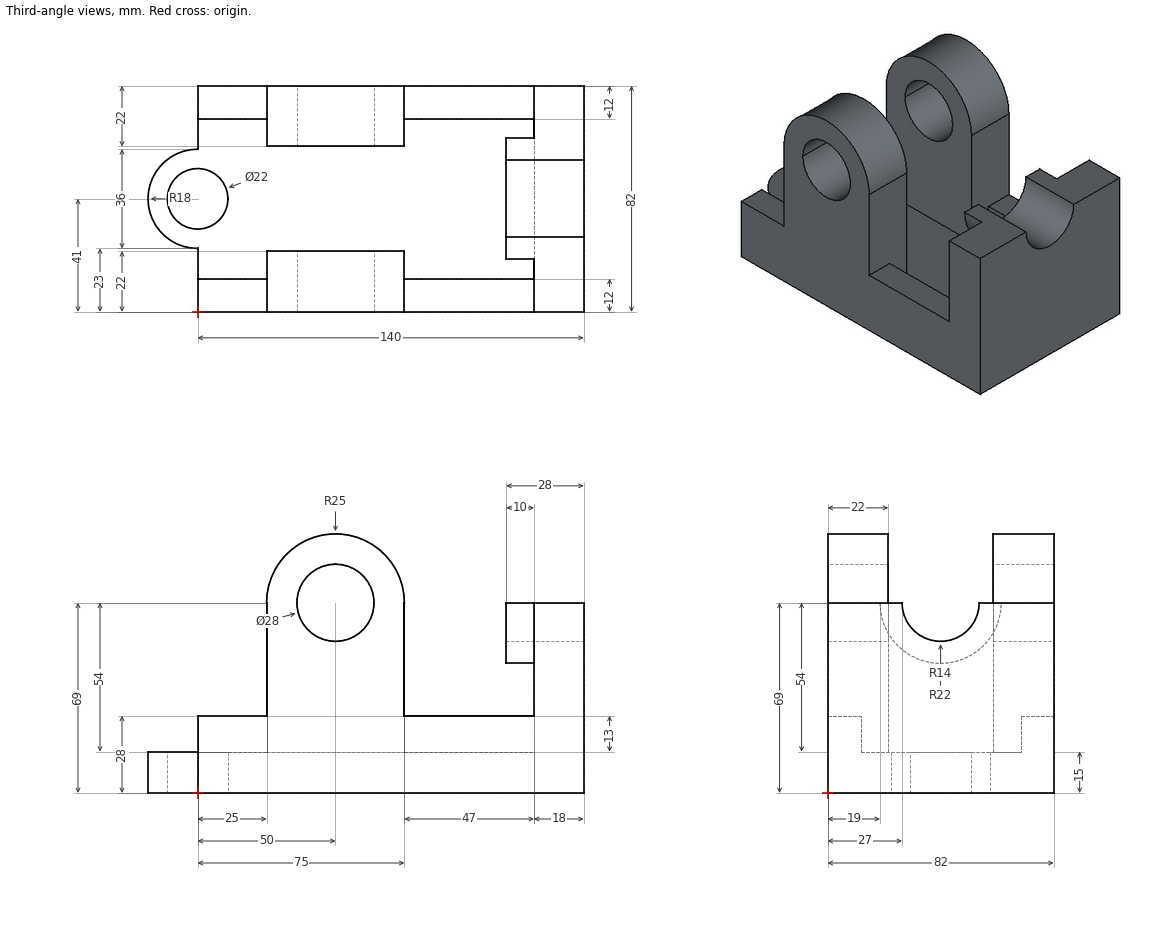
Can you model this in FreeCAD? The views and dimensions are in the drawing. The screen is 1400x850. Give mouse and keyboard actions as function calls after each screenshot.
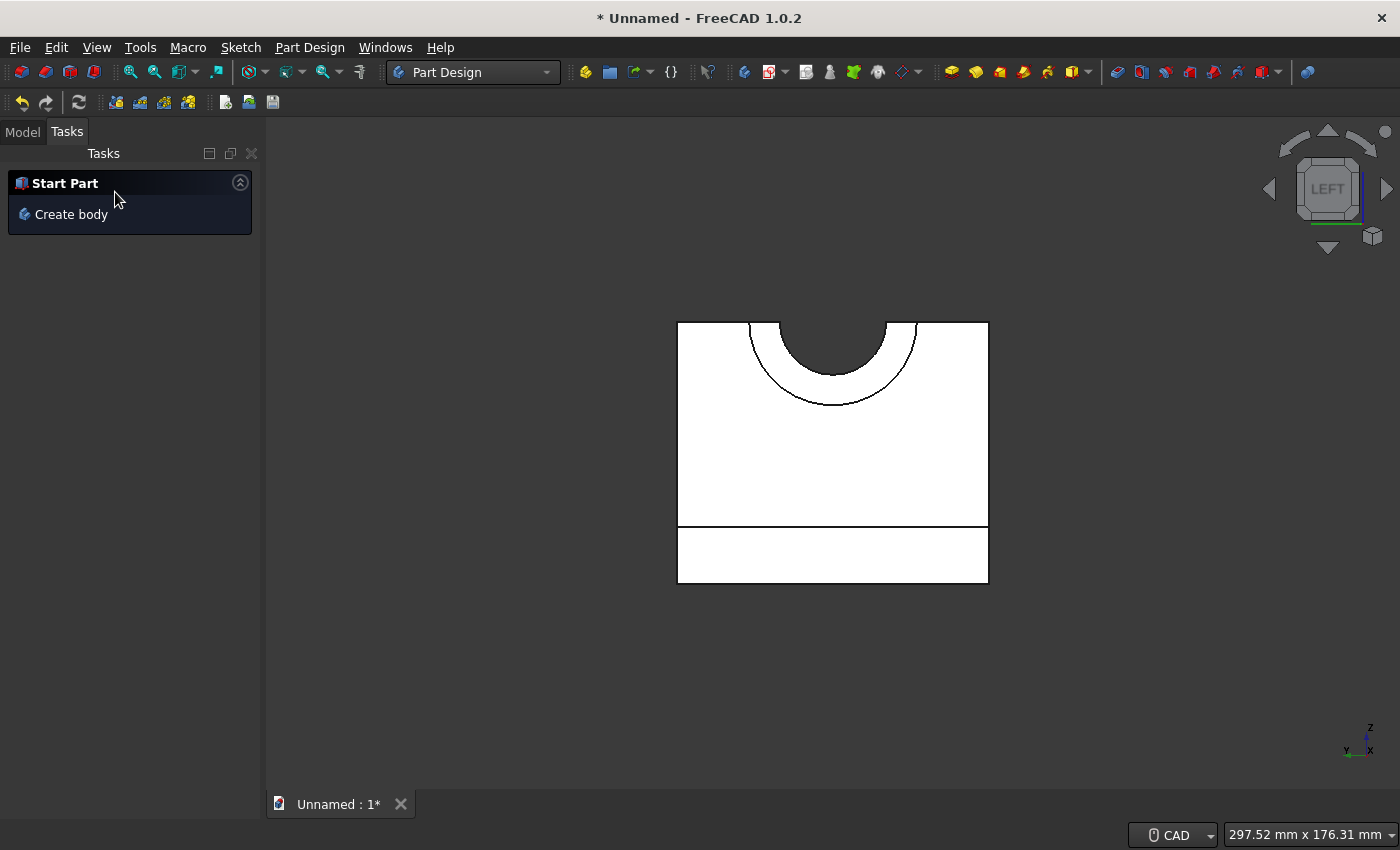
click(132, 72)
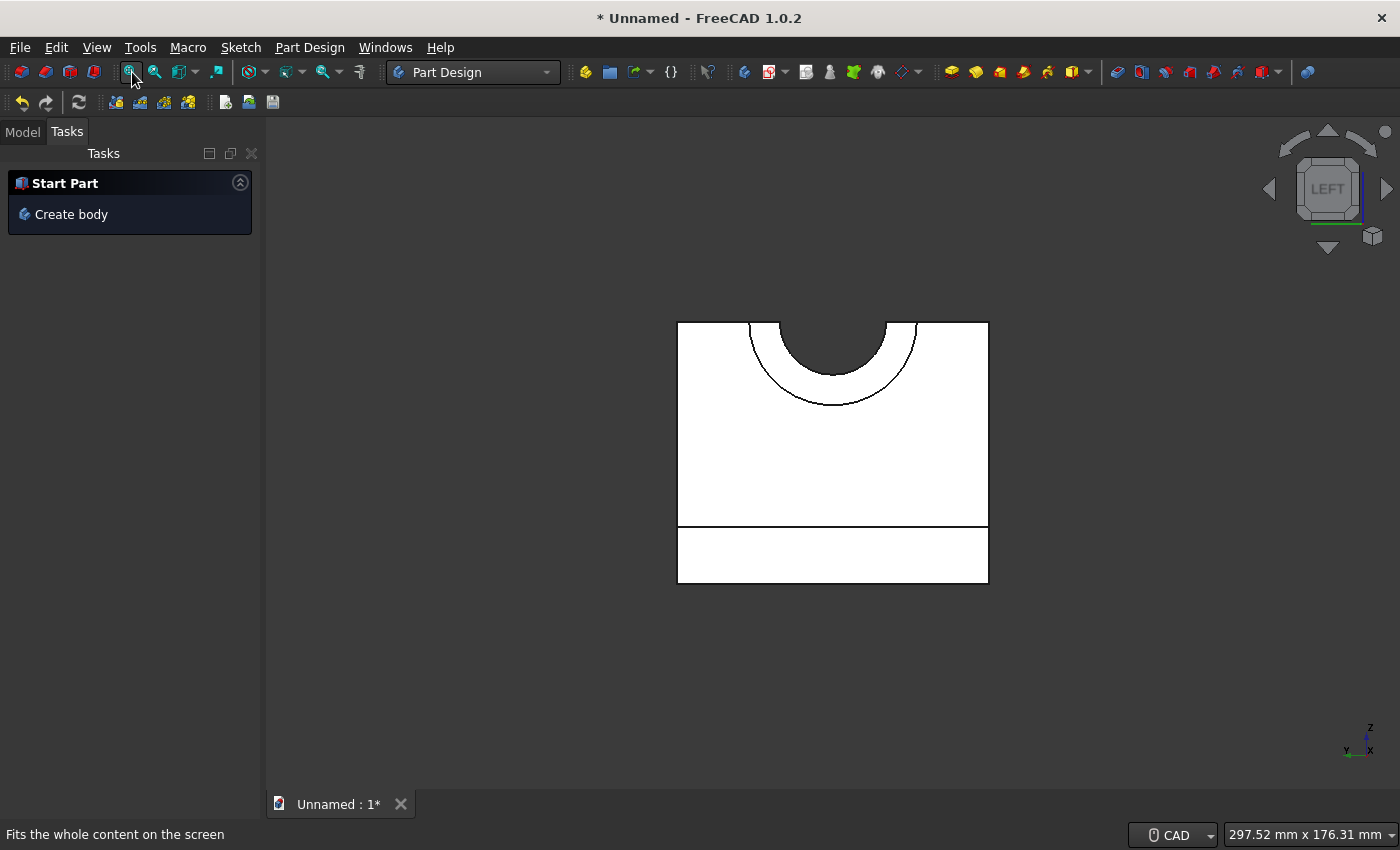
click(770, 72)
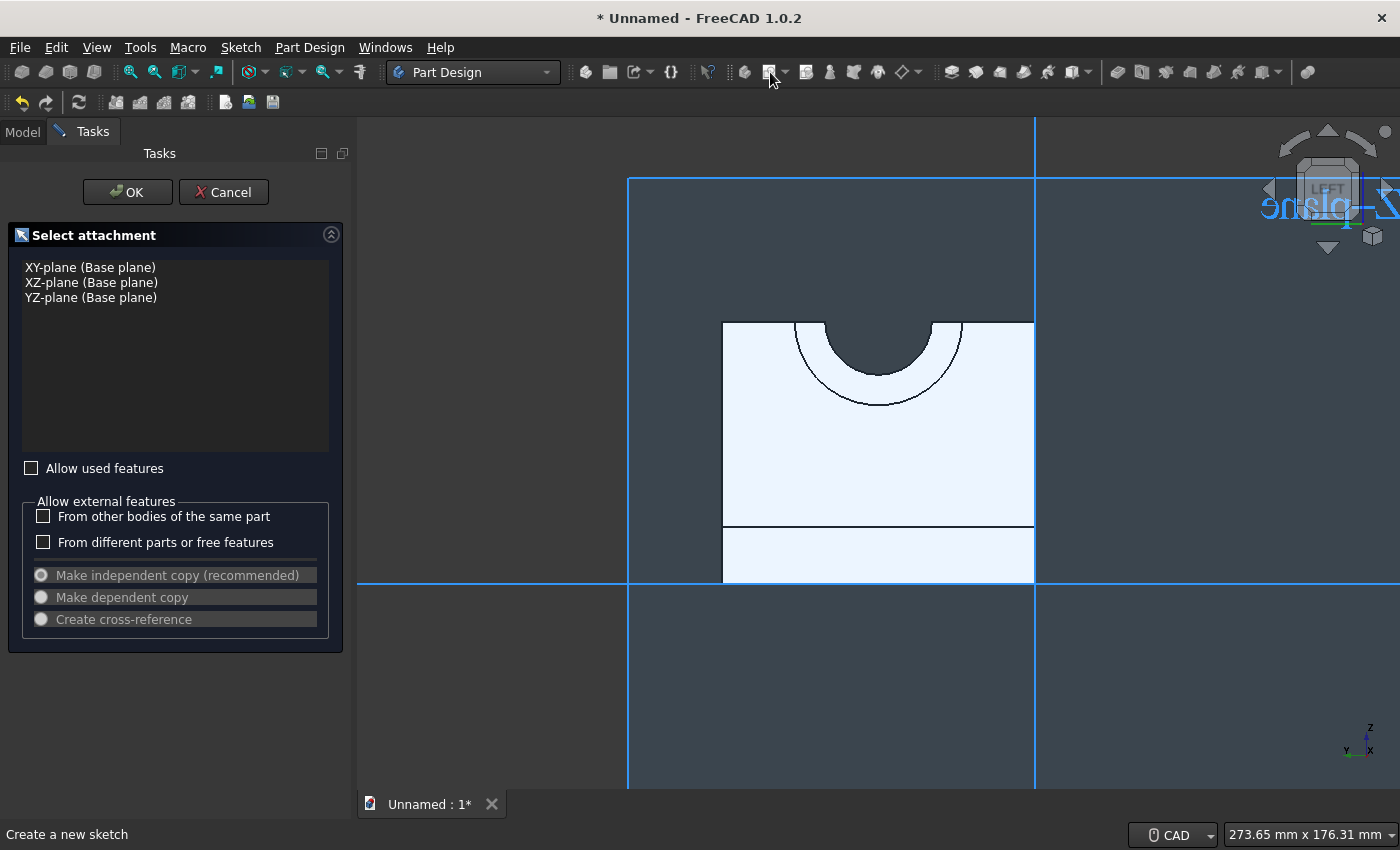
click(82, 282)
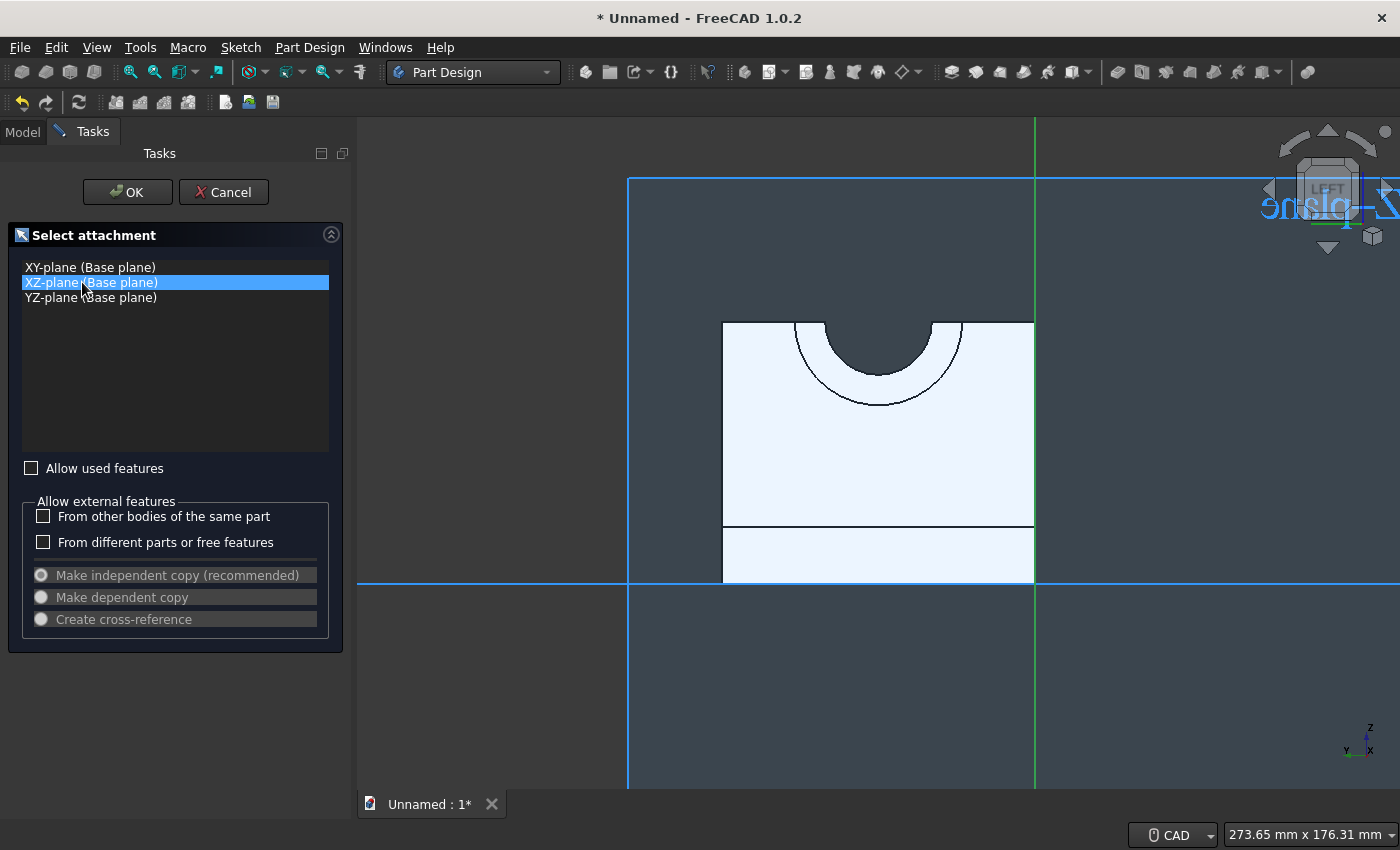
click(128, 192)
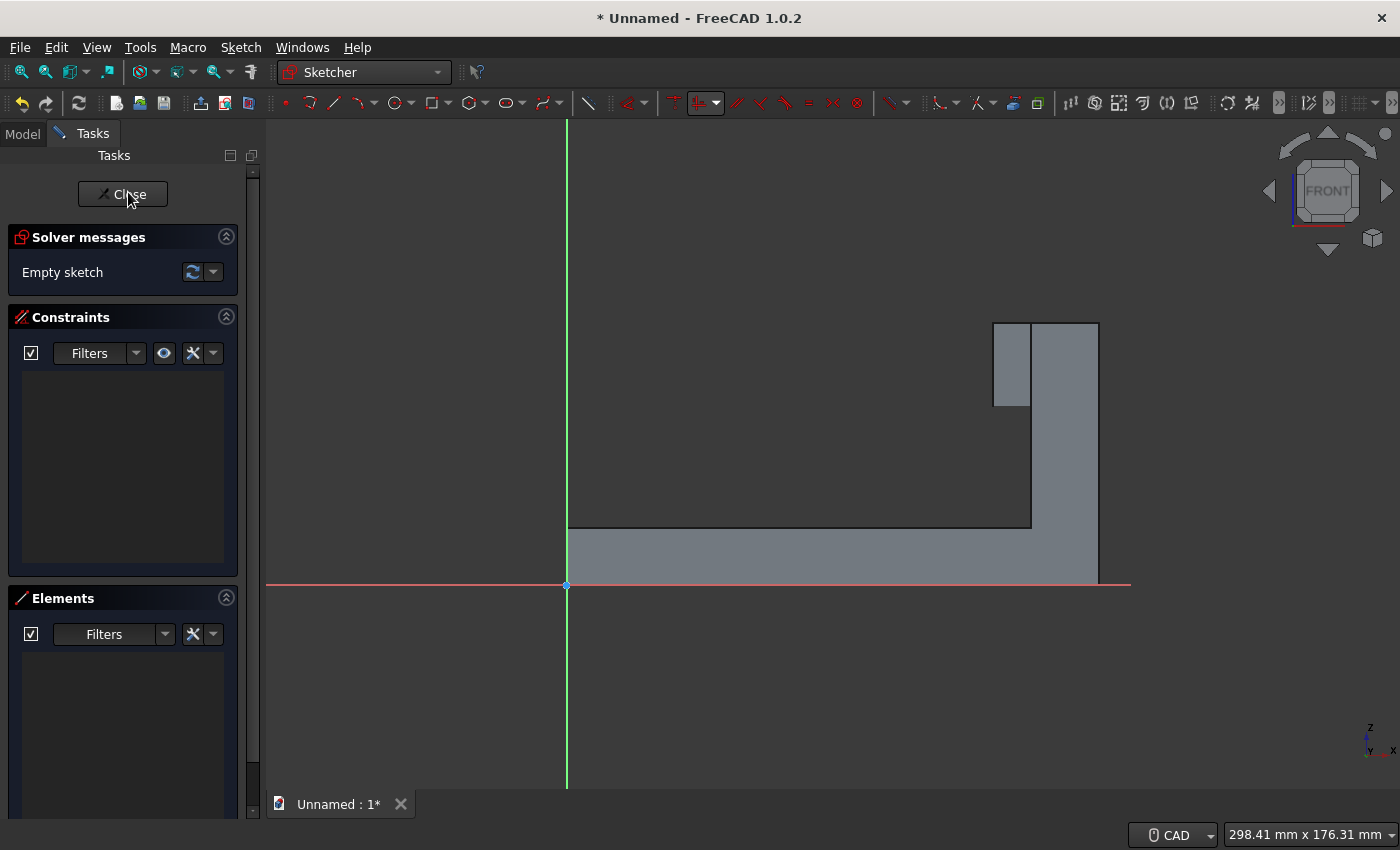
click(310, 104)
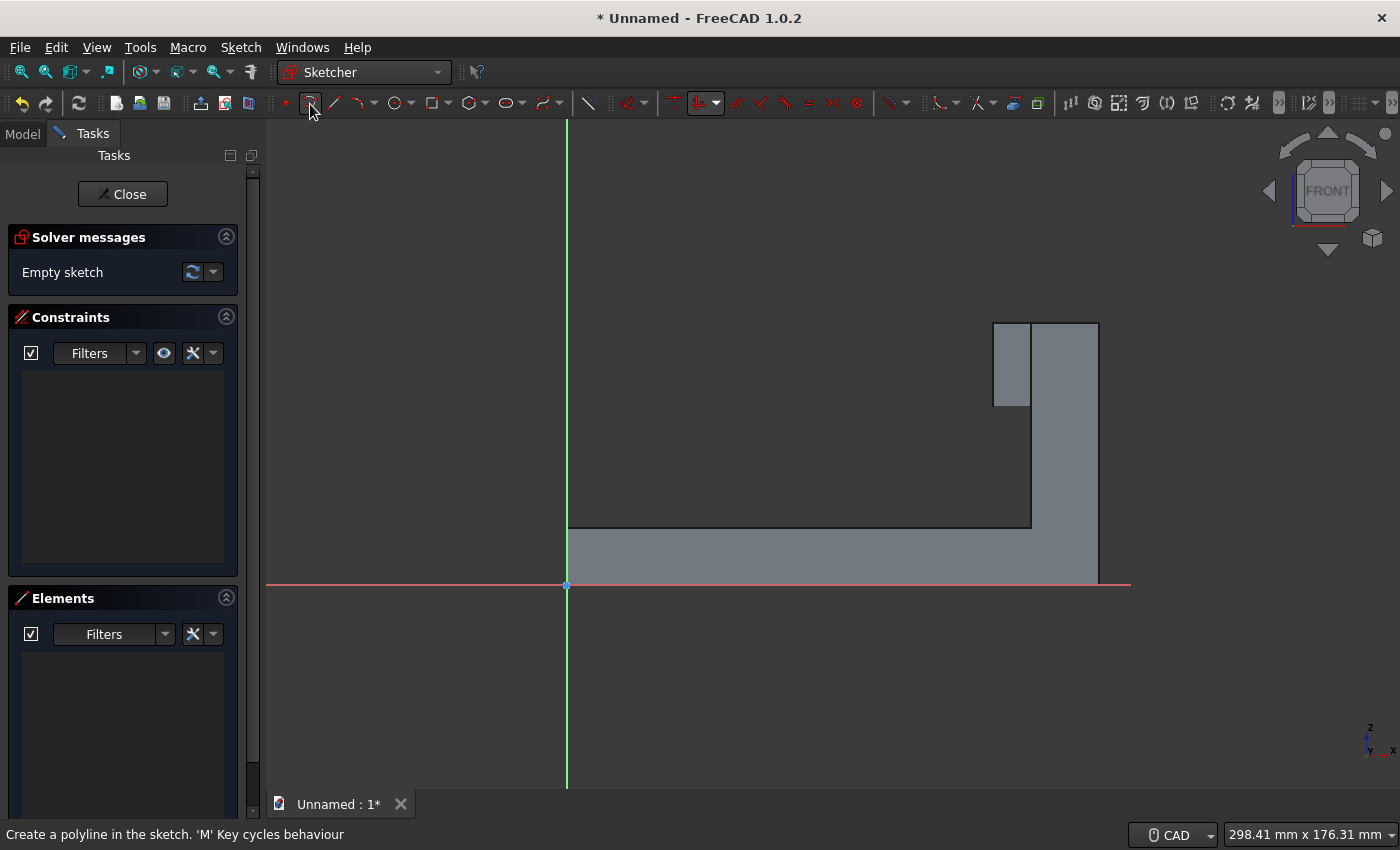
click(662, 323)
click(662, 528)
click(852, 528)
click(852, 323)
right_click(852, 323)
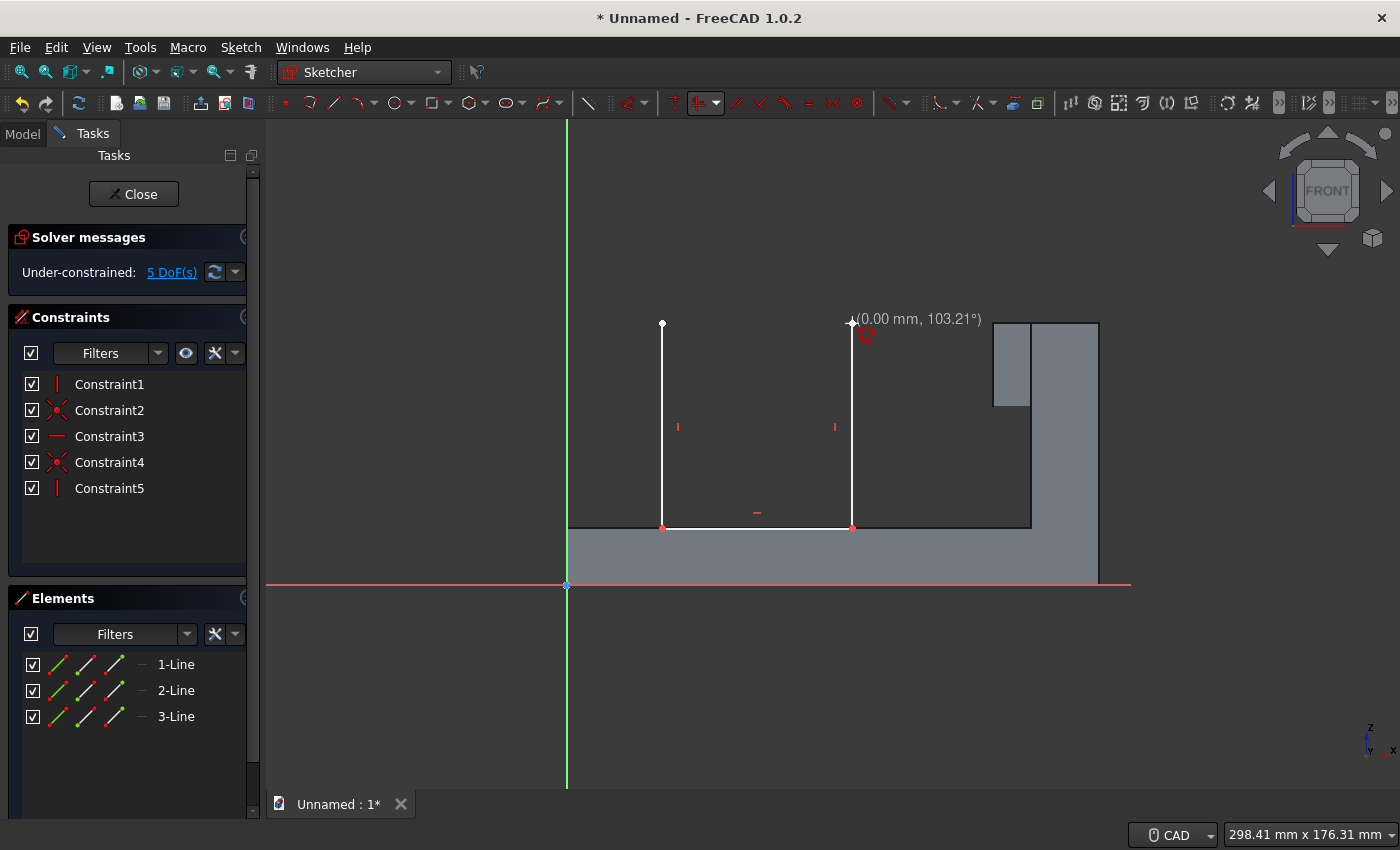
click(358, 104)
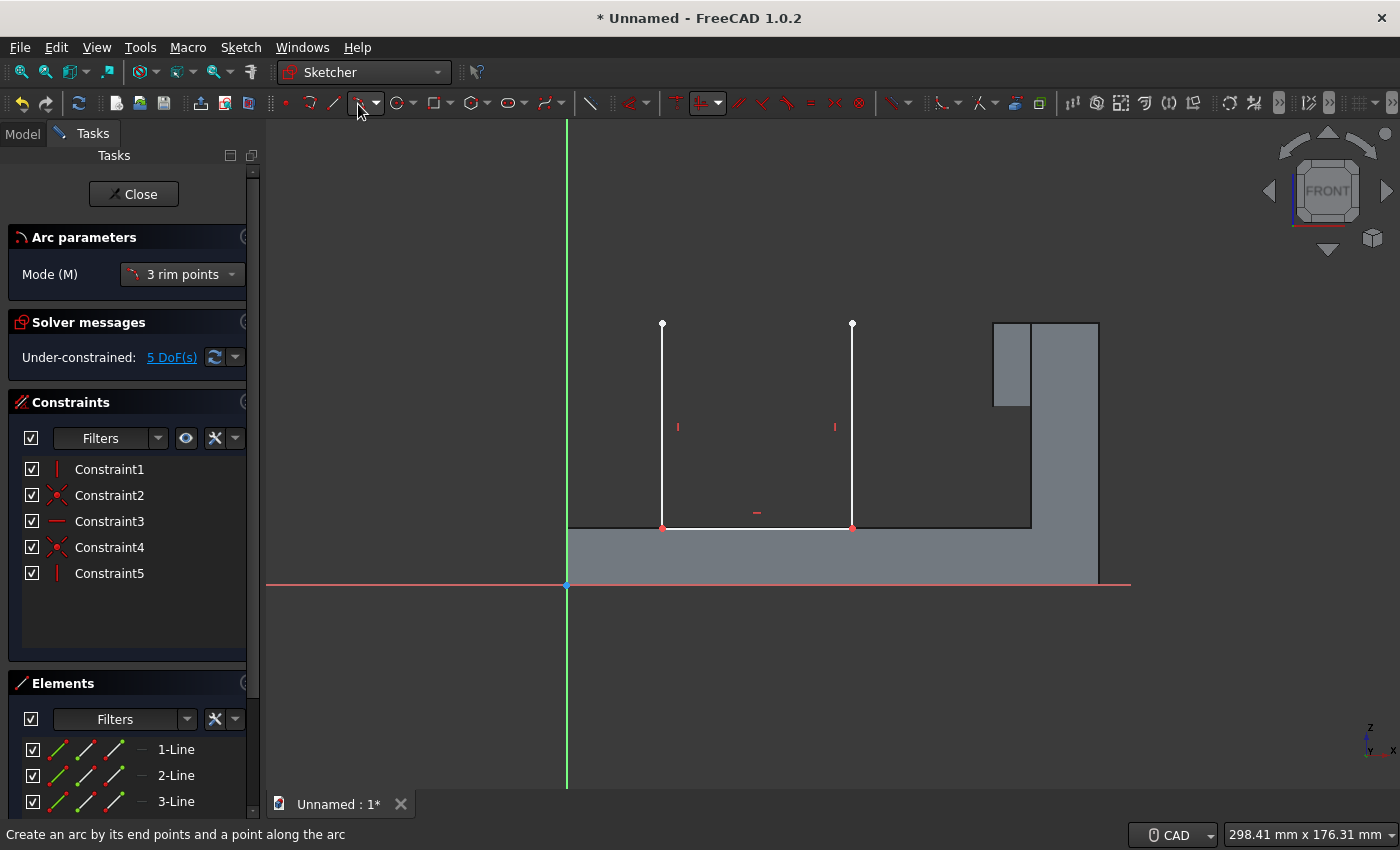
click(852, 324)
click(662, 324)
click(757, 228)
key(Escape)